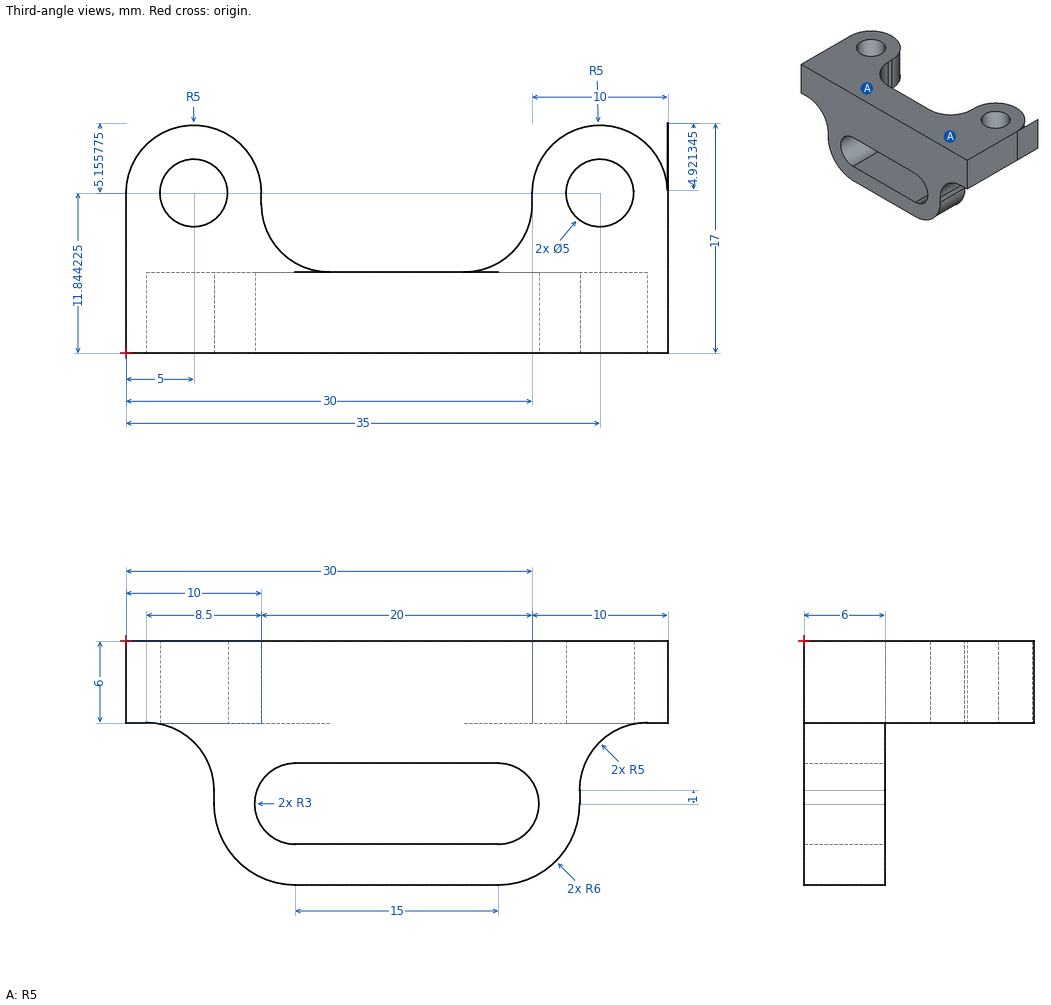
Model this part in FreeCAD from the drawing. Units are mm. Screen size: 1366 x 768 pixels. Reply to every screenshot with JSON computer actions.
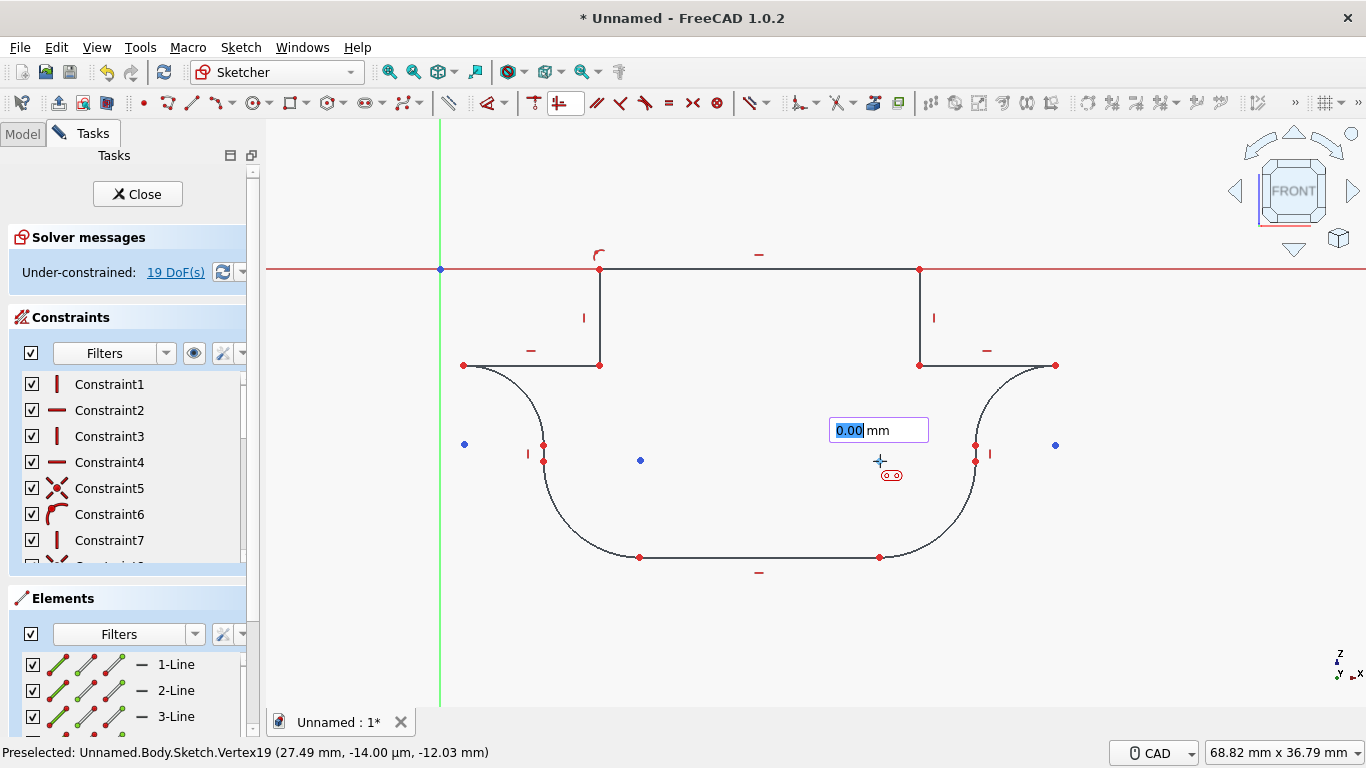
{"action": "left_click", "coordinate": [760, 413]}
{"action": "key", "text": "Escape"}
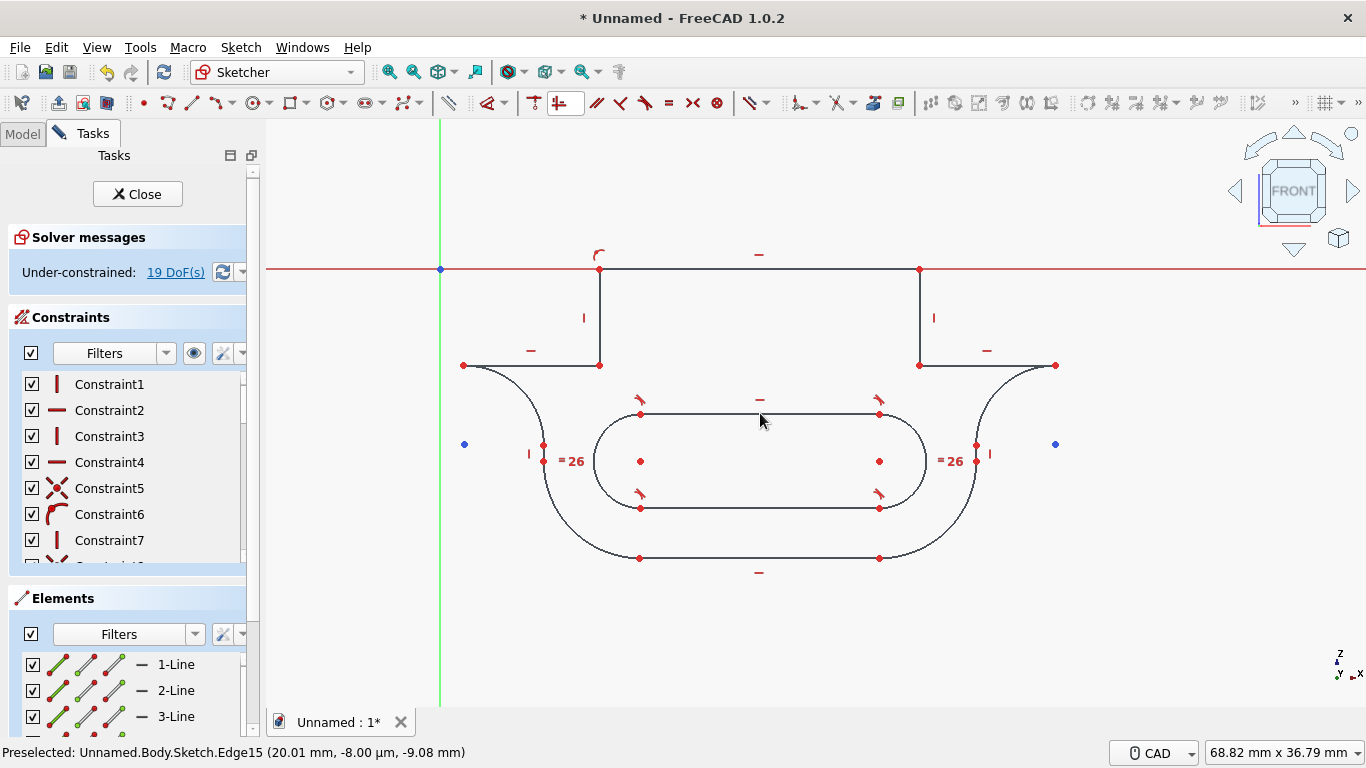
{"action": "scroll", "coordinate": [976, 454], "scroll_direction": "up", "scroll_amount": 3}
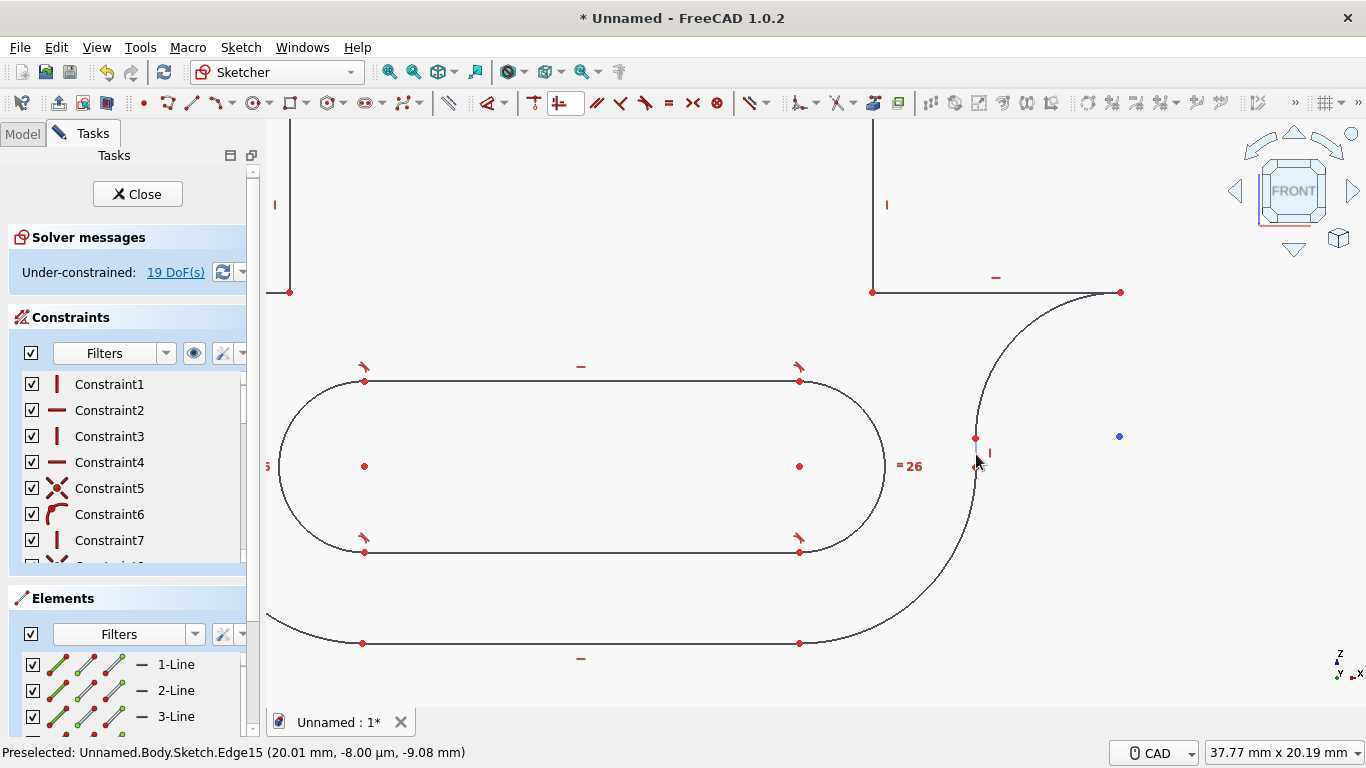
{"action": "left_click", "coordinate": [976, 453]}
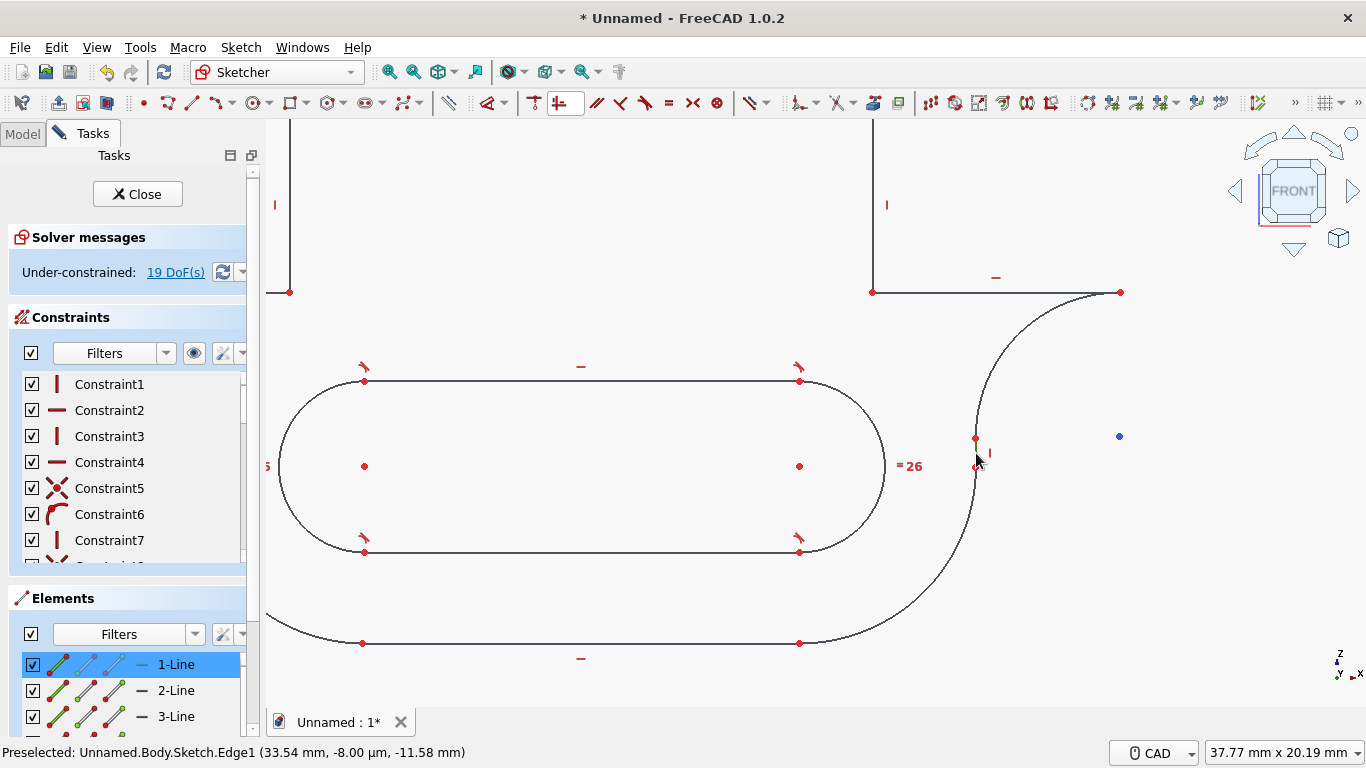
{"action": "left_click", "coordinate": [880, 624]}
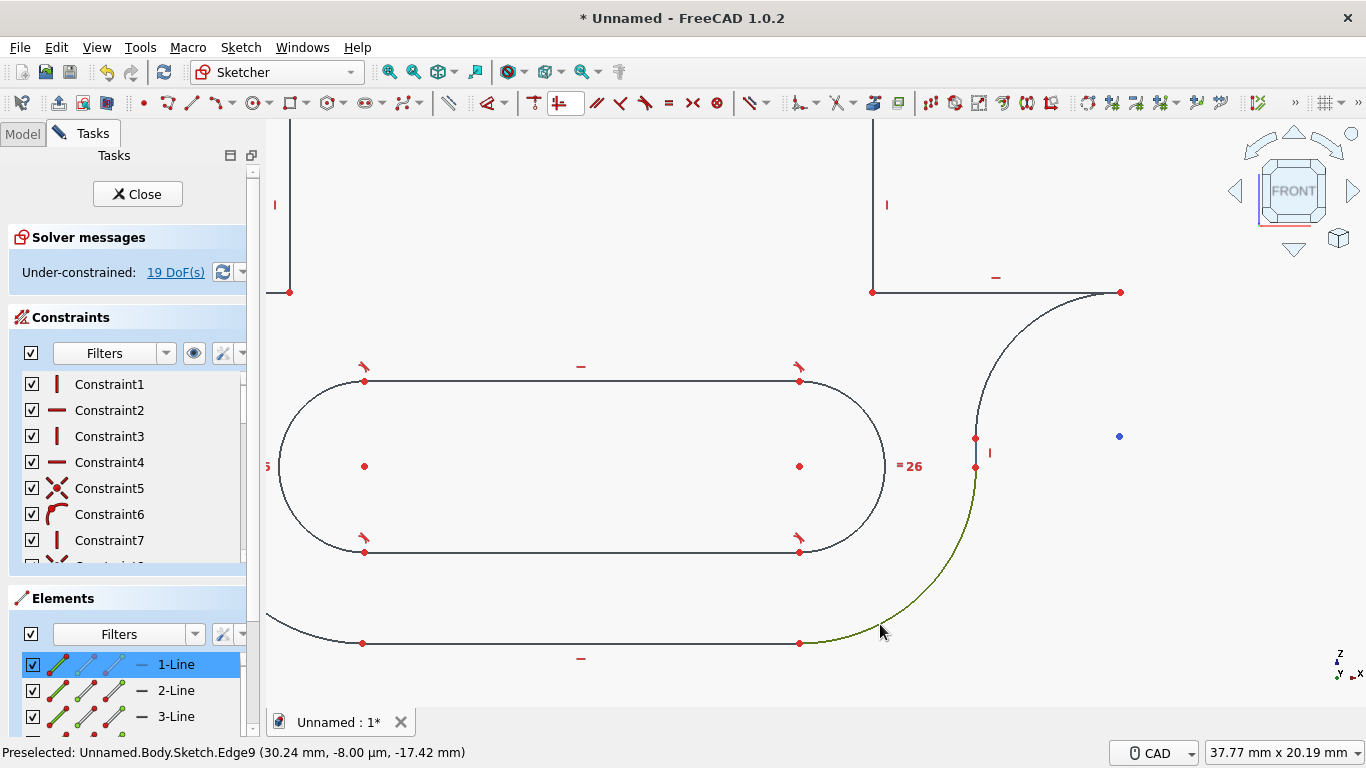
{"action": "left_click", "coordinate": [646, 104]}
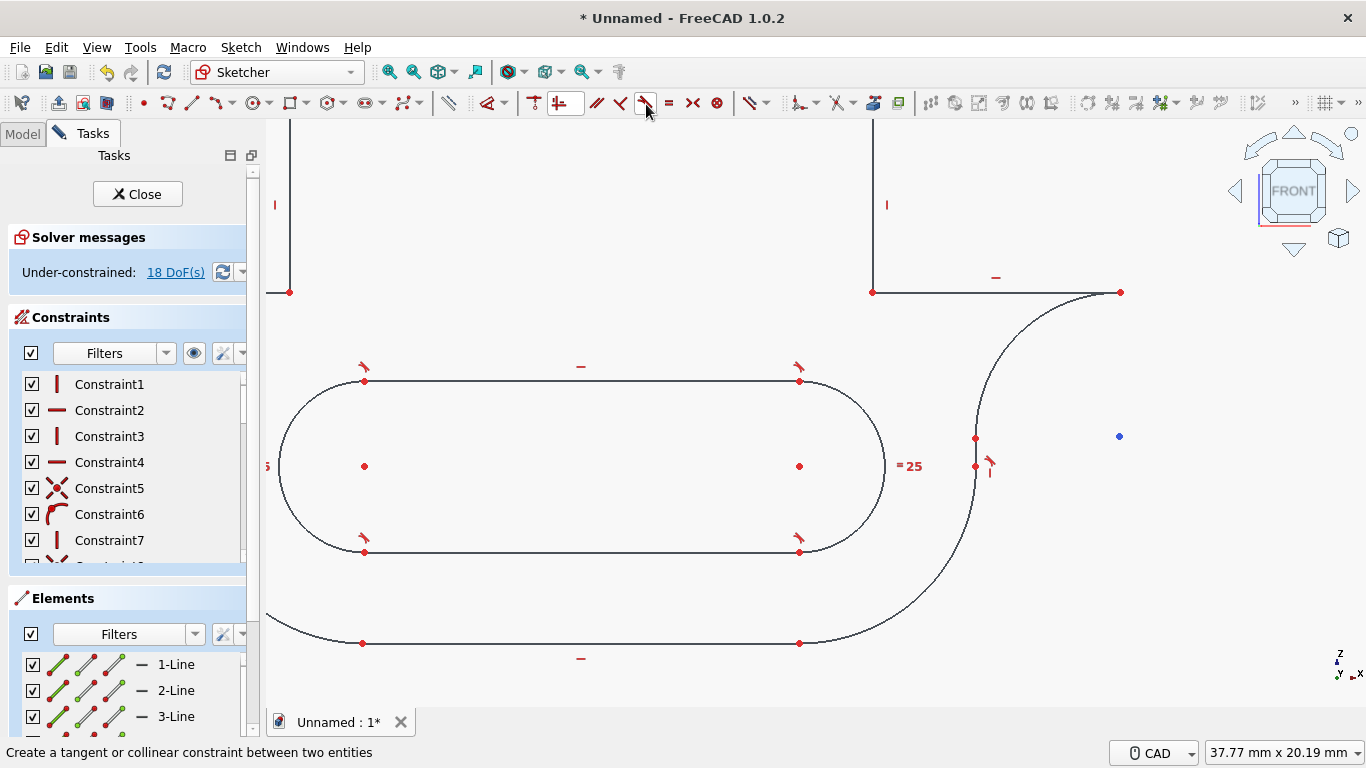
{"action": "left_click", "coordinate": [976, 450]}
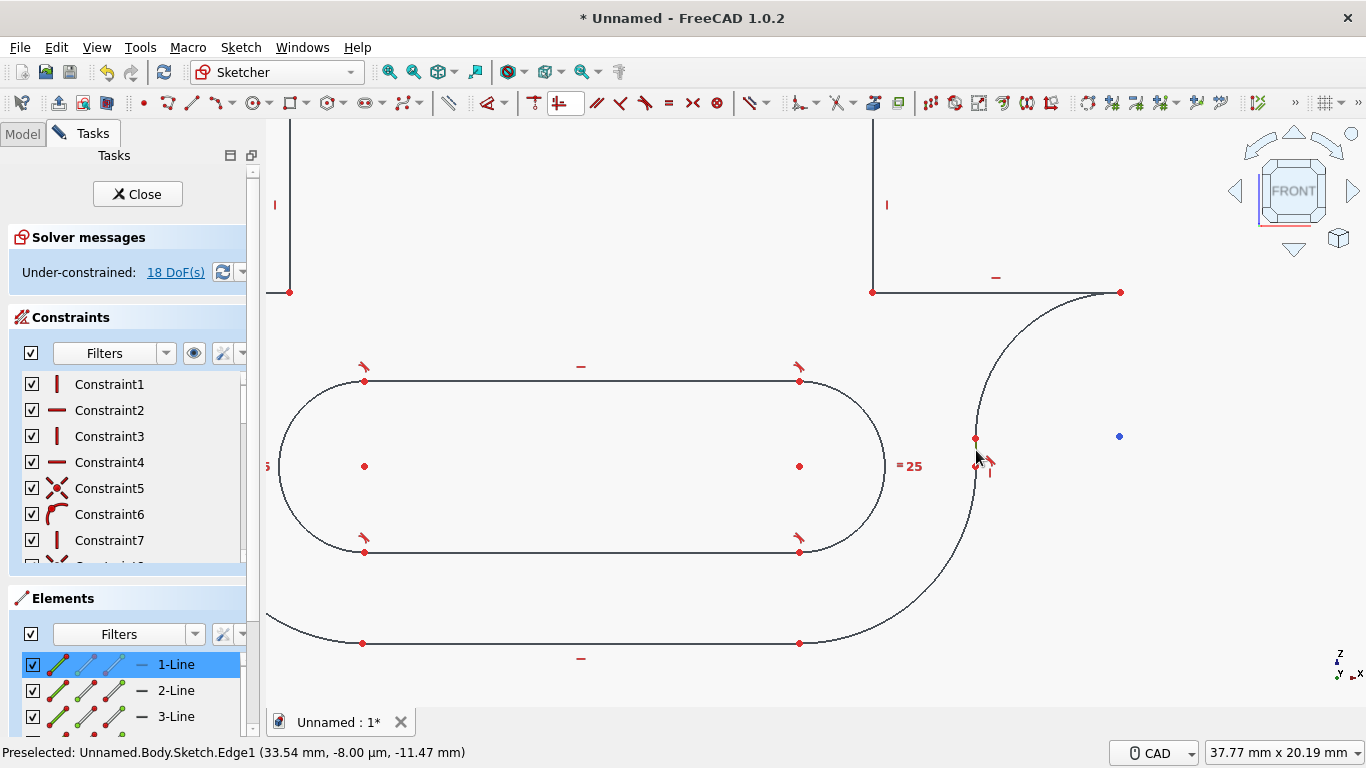
{"action": "left_click", "coordinate": [1055, 308]}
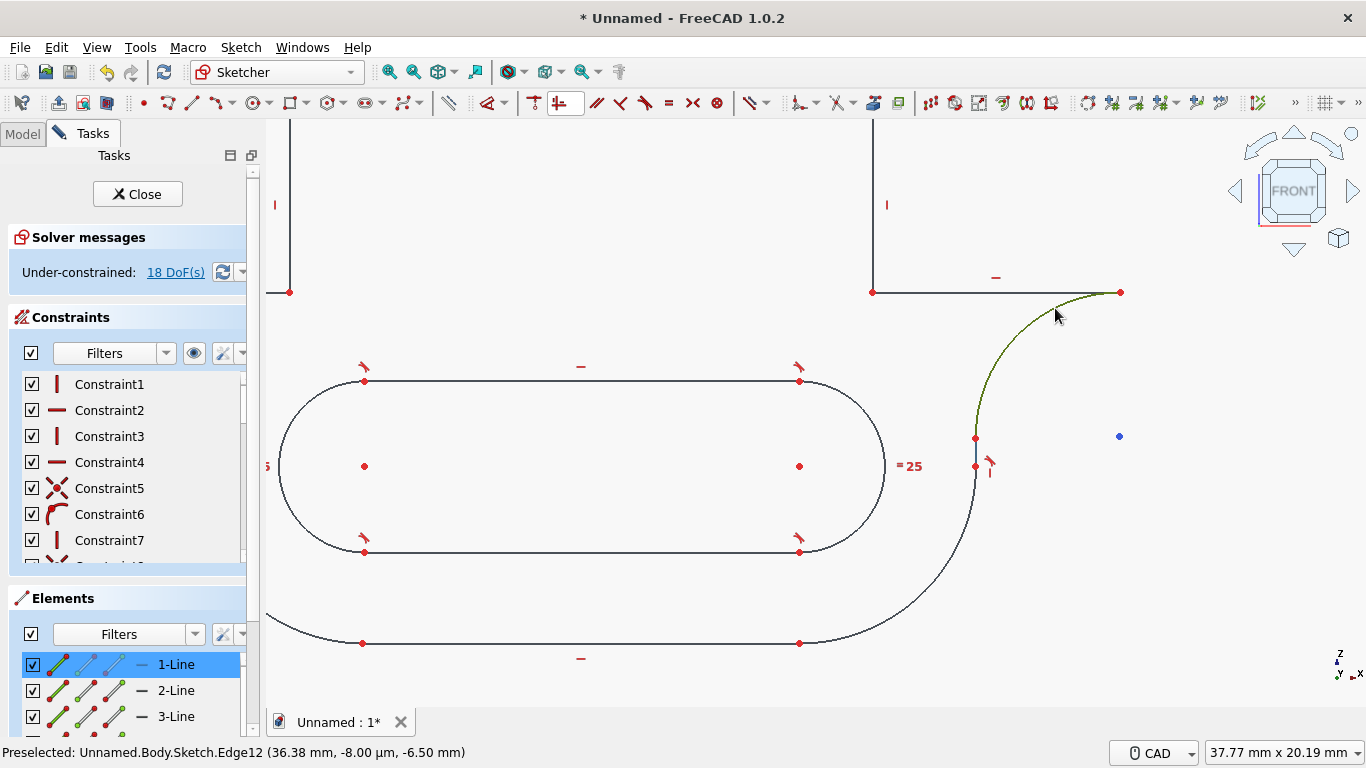
{"action": "left_click", "coordinate": [646, 104]}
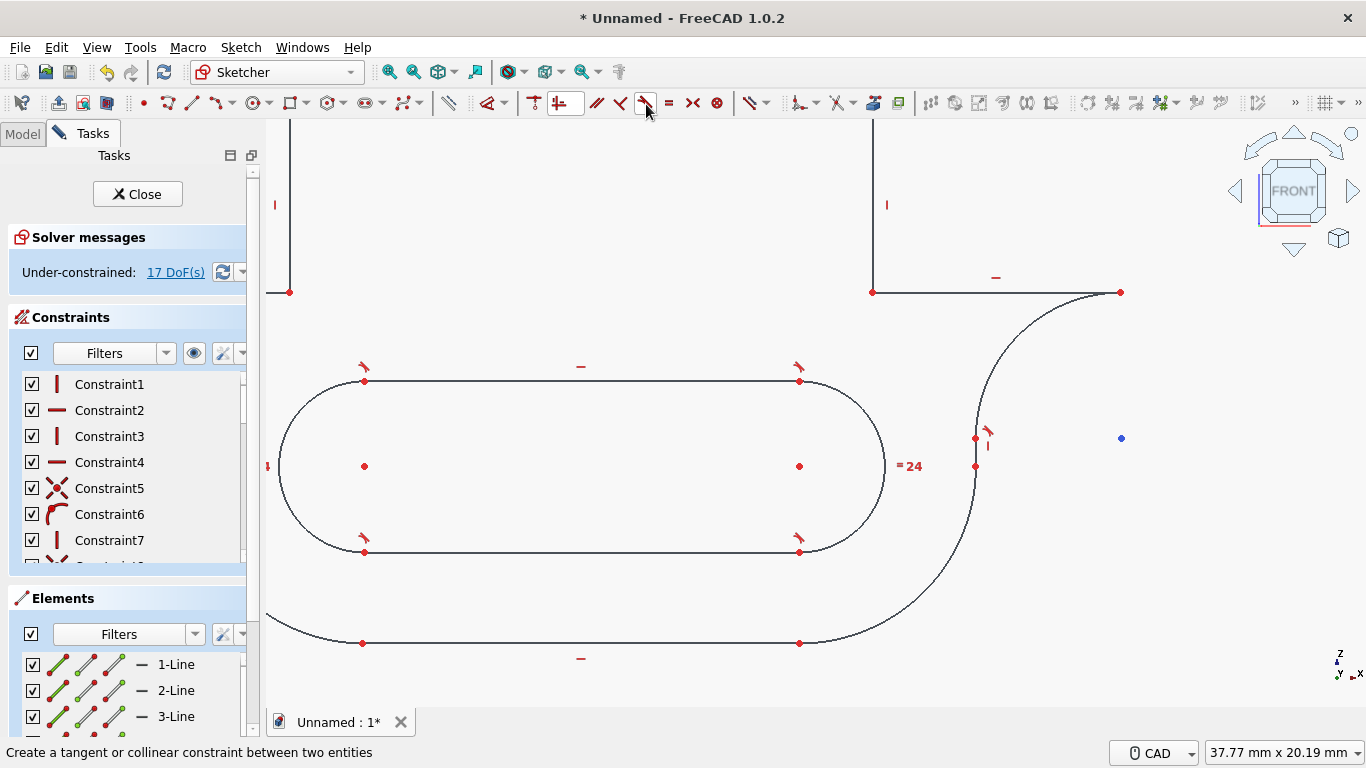
{"action": "left_click", "coordinate": [669, 643]}